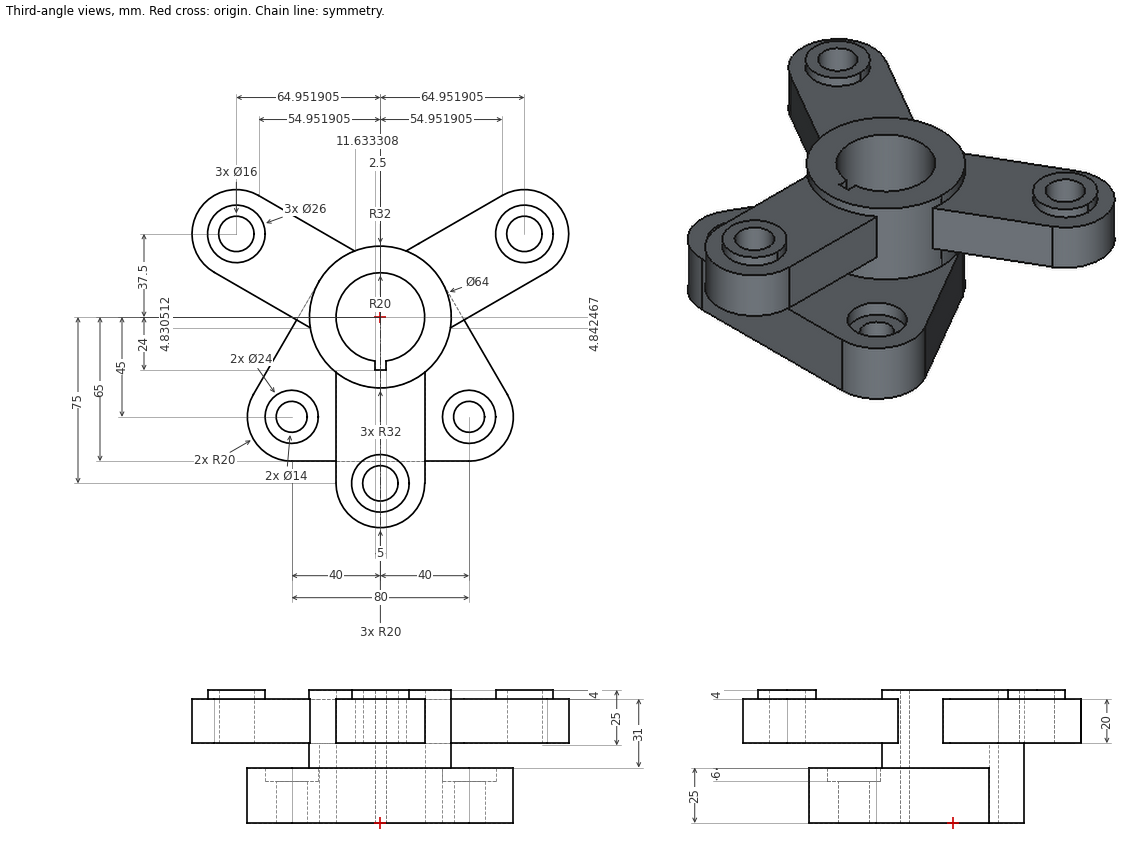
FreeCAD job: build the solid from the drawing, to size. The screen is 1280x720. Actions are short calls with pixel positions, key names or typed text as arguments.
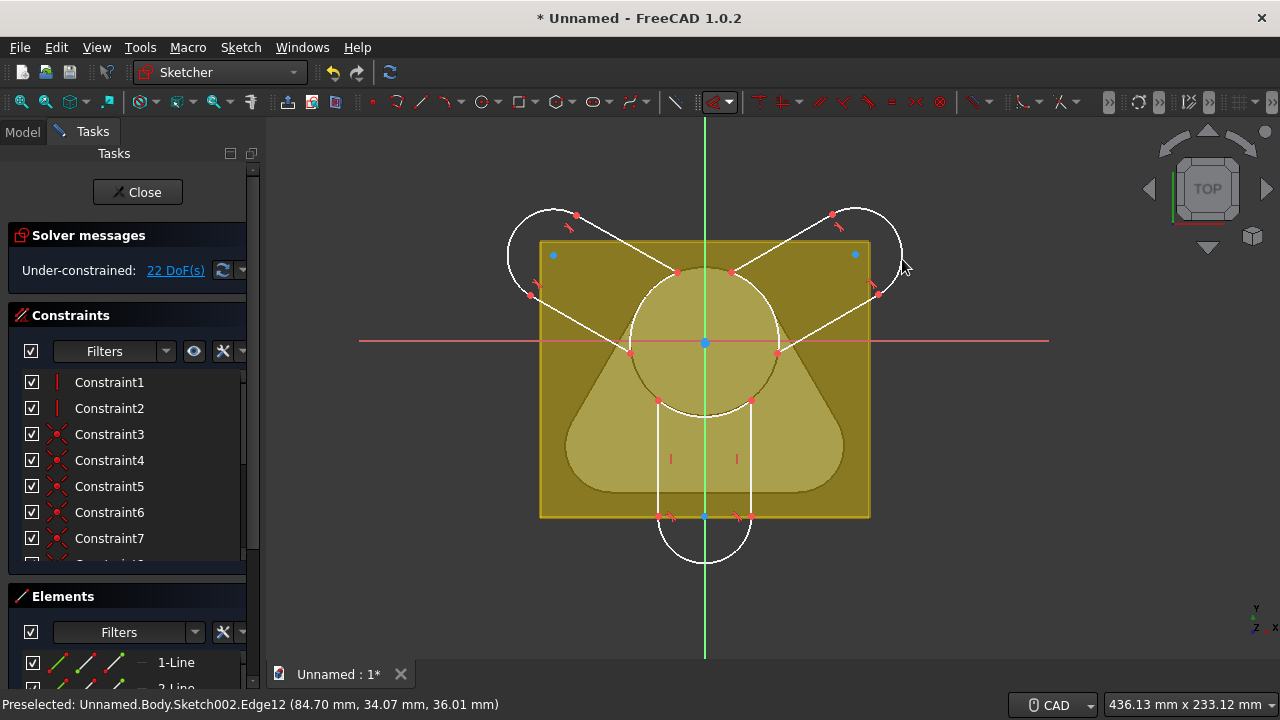
click(685, 414)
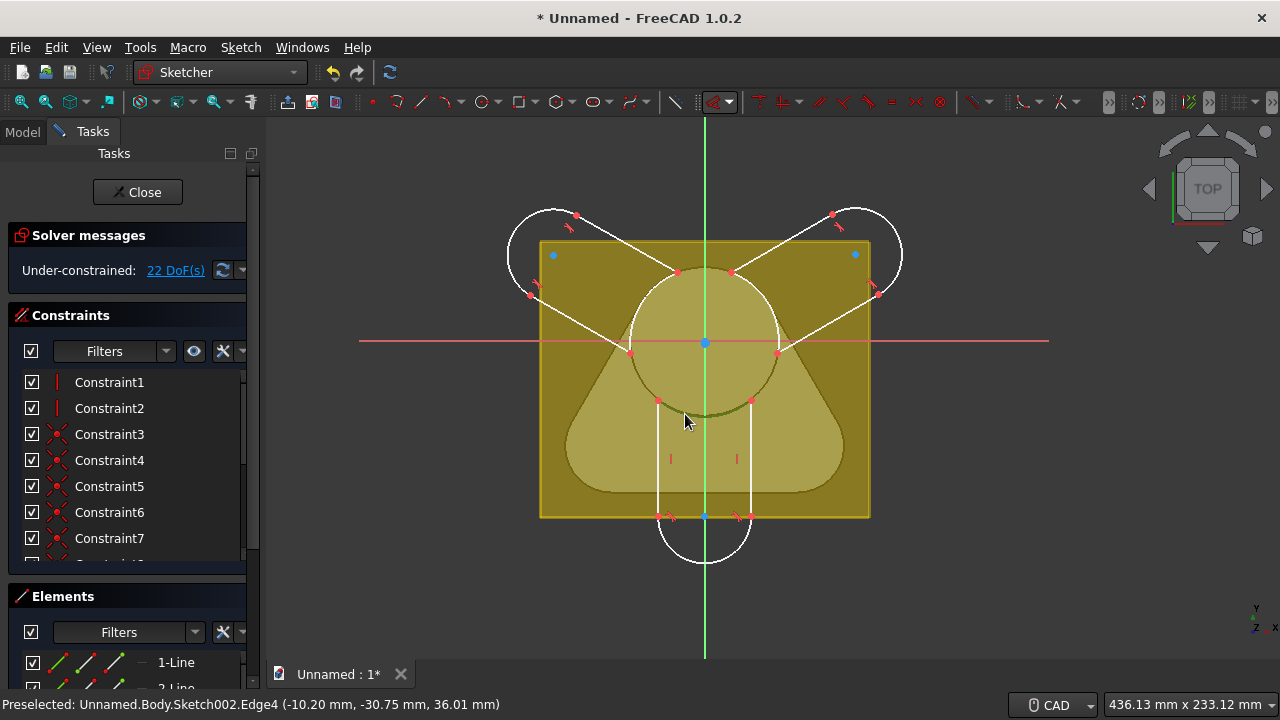
click(653, 289)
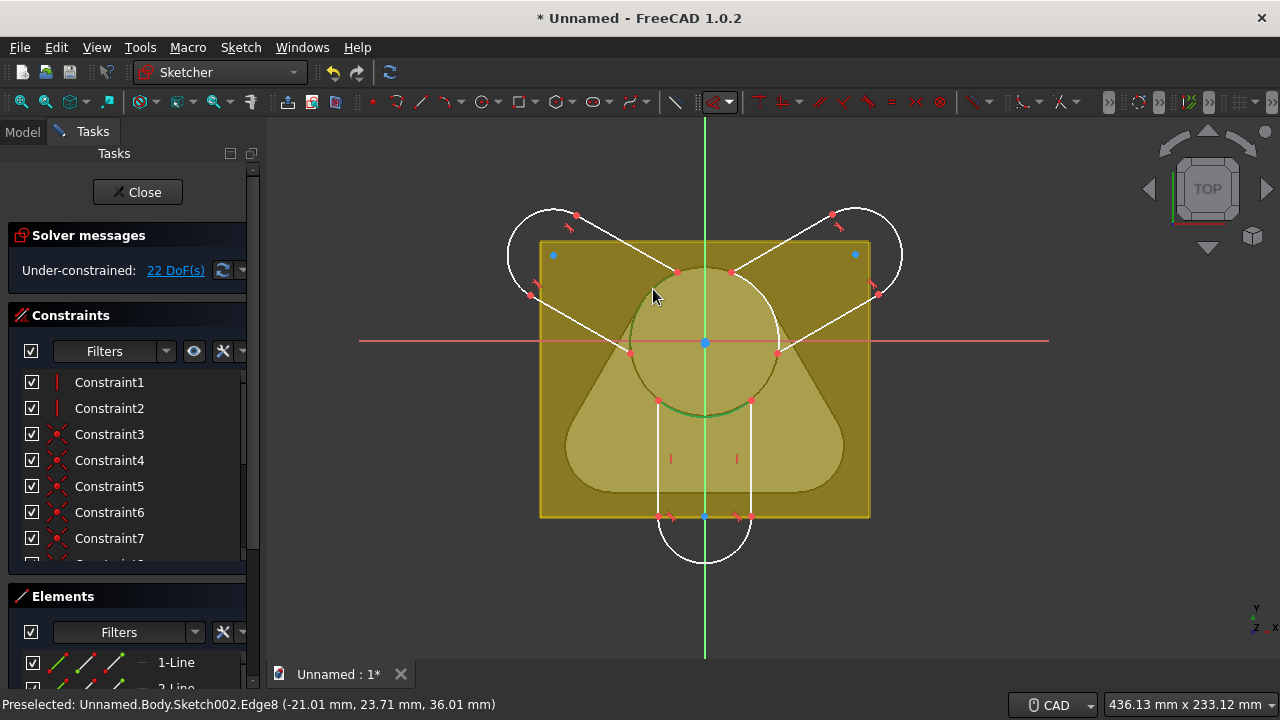
key(c)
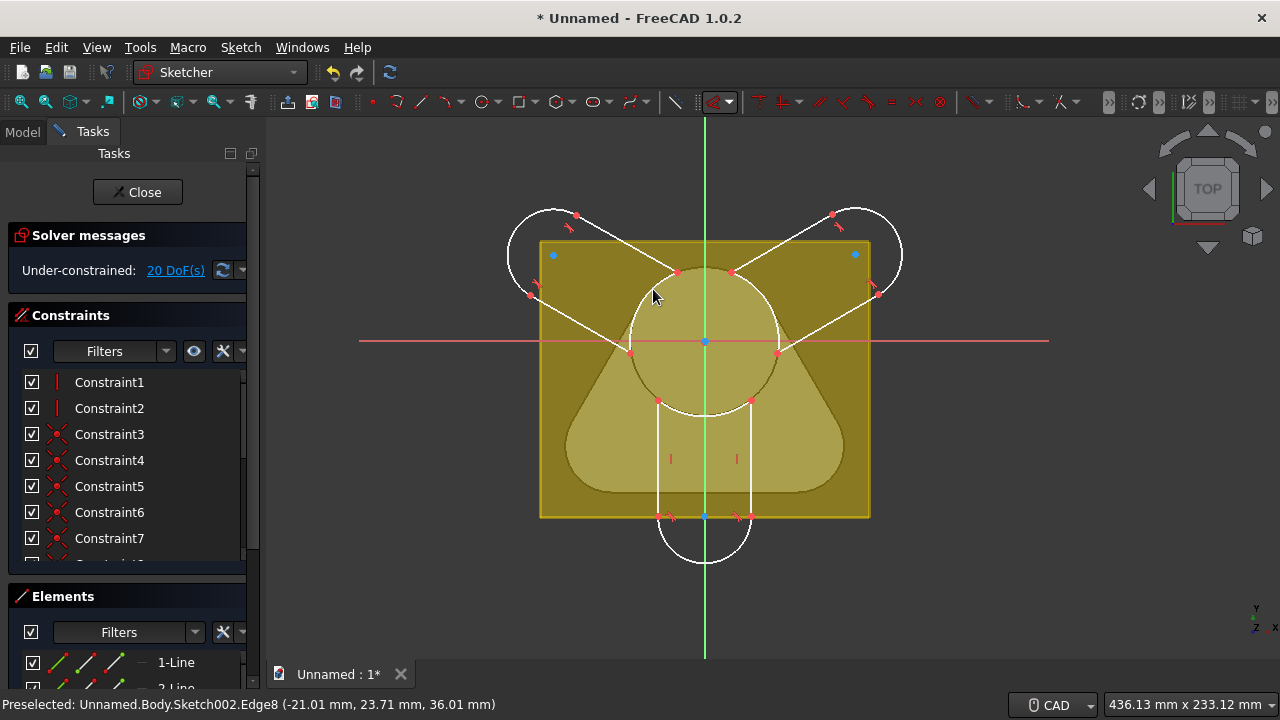
click(685, 414)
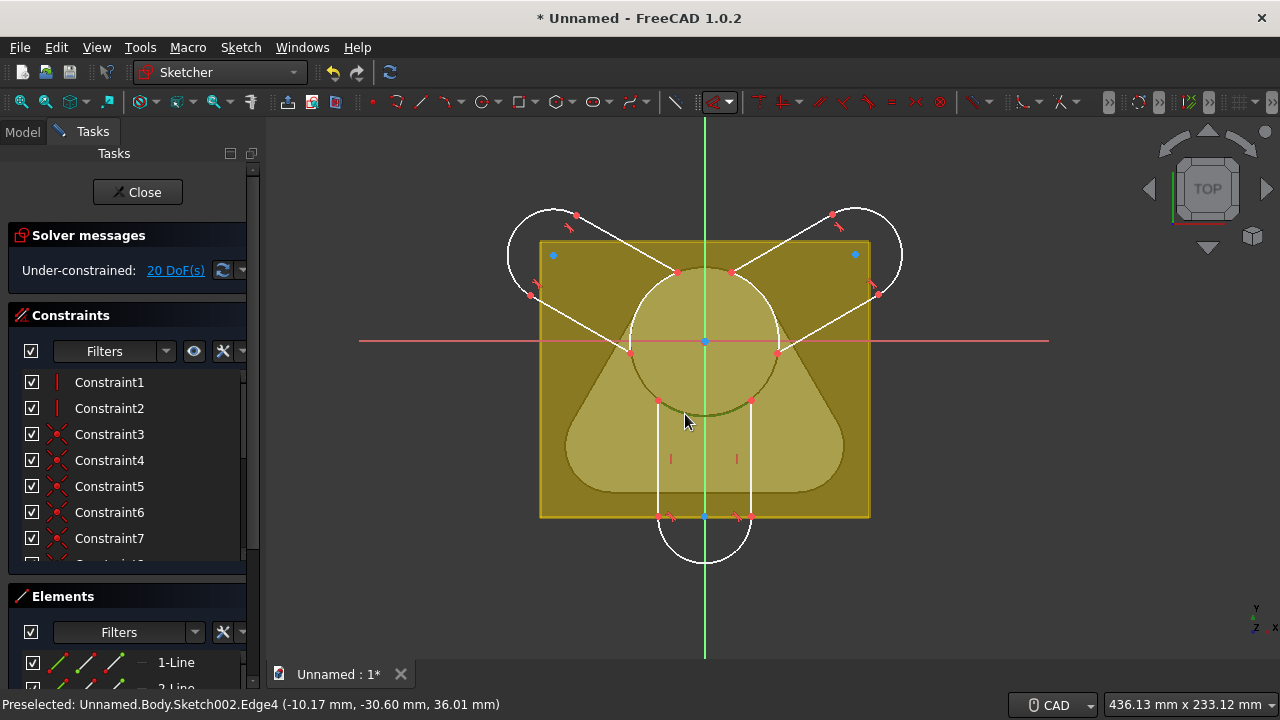
click(777, 323)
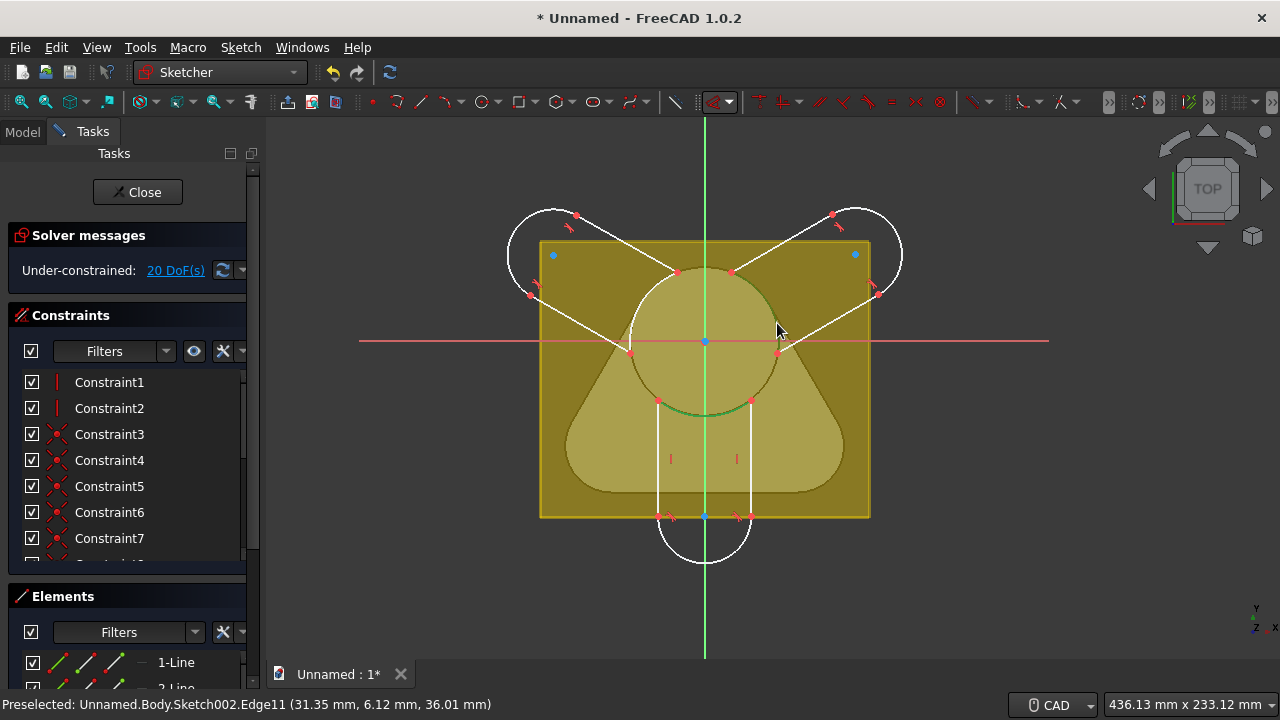
key(c)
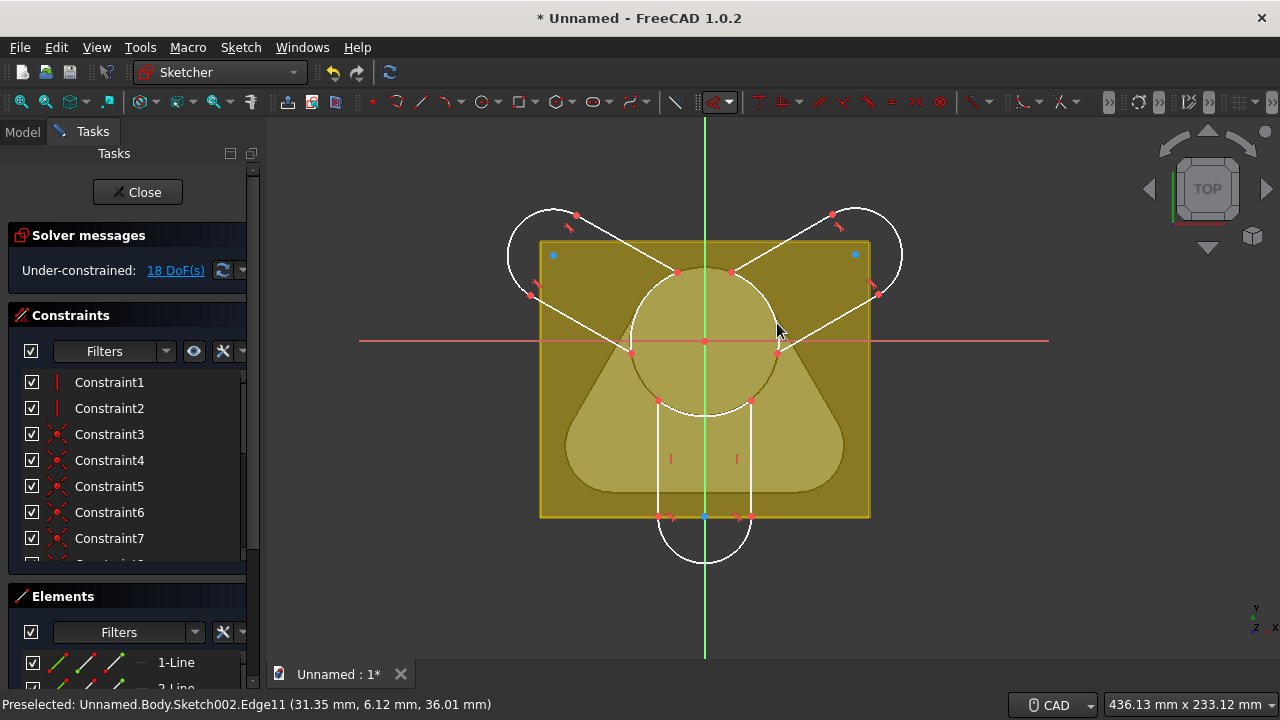
drag(695, 331, 715, 352)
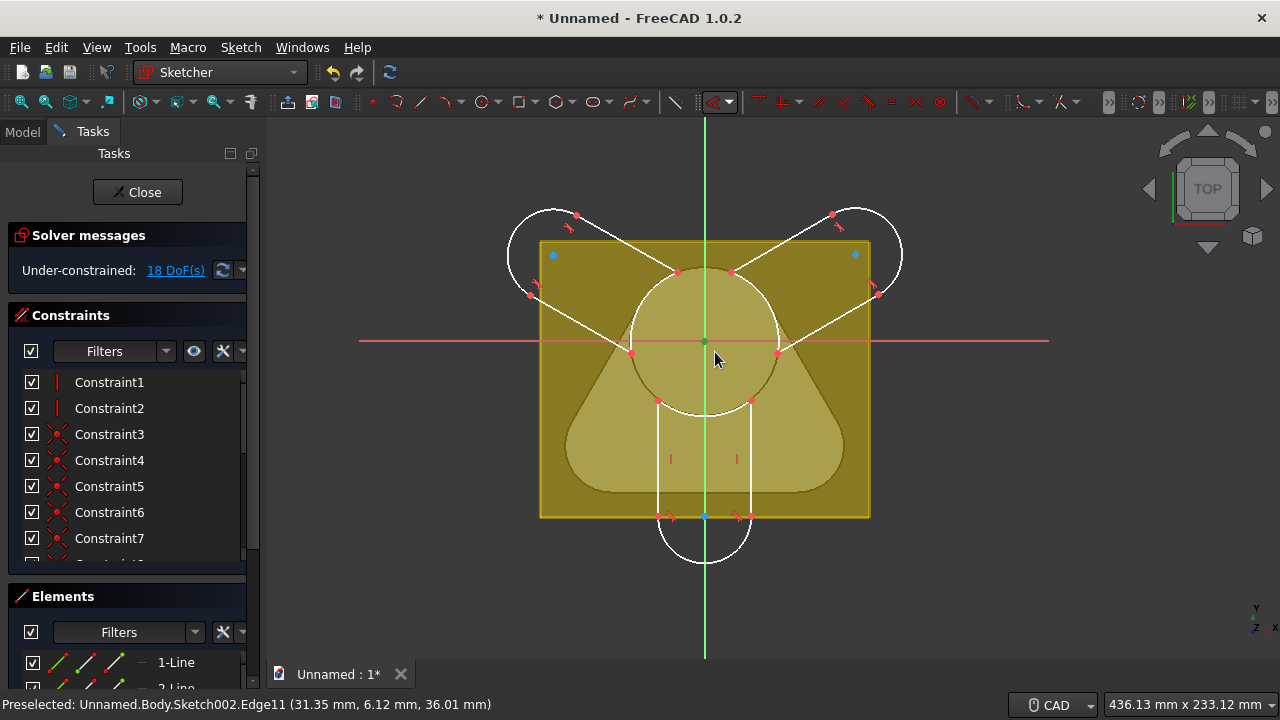
key(c)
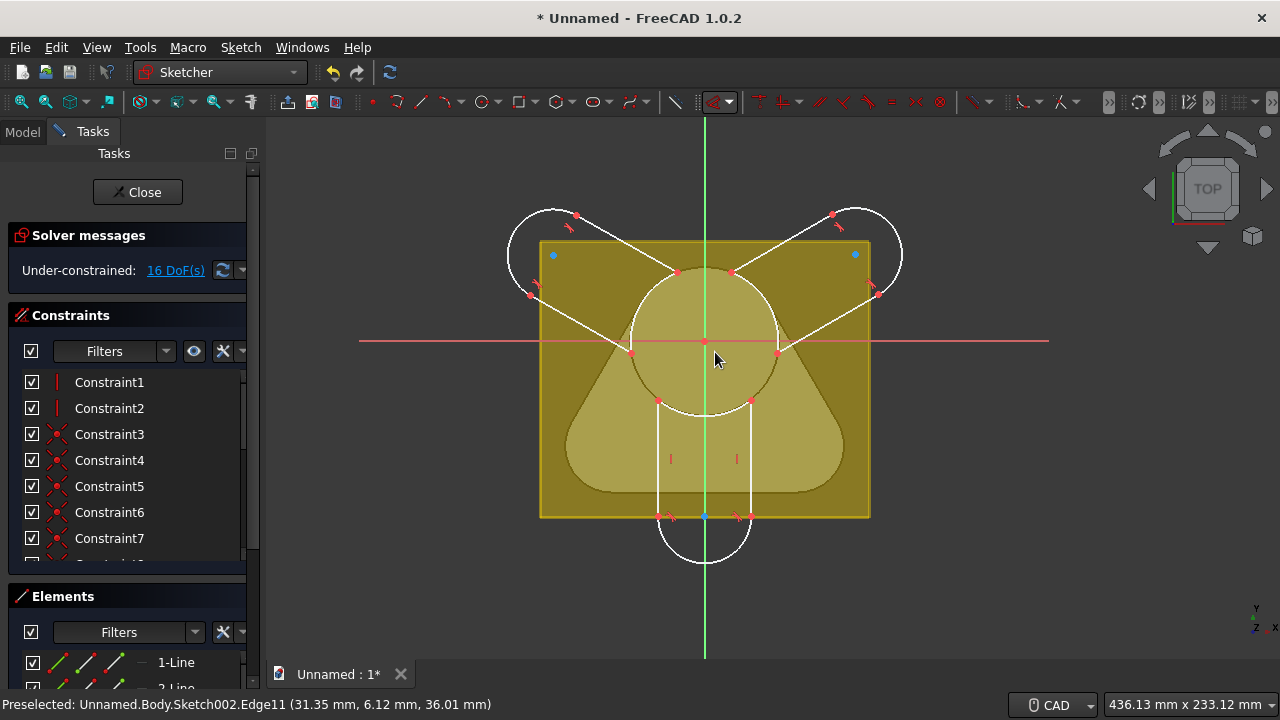
click(677, 554)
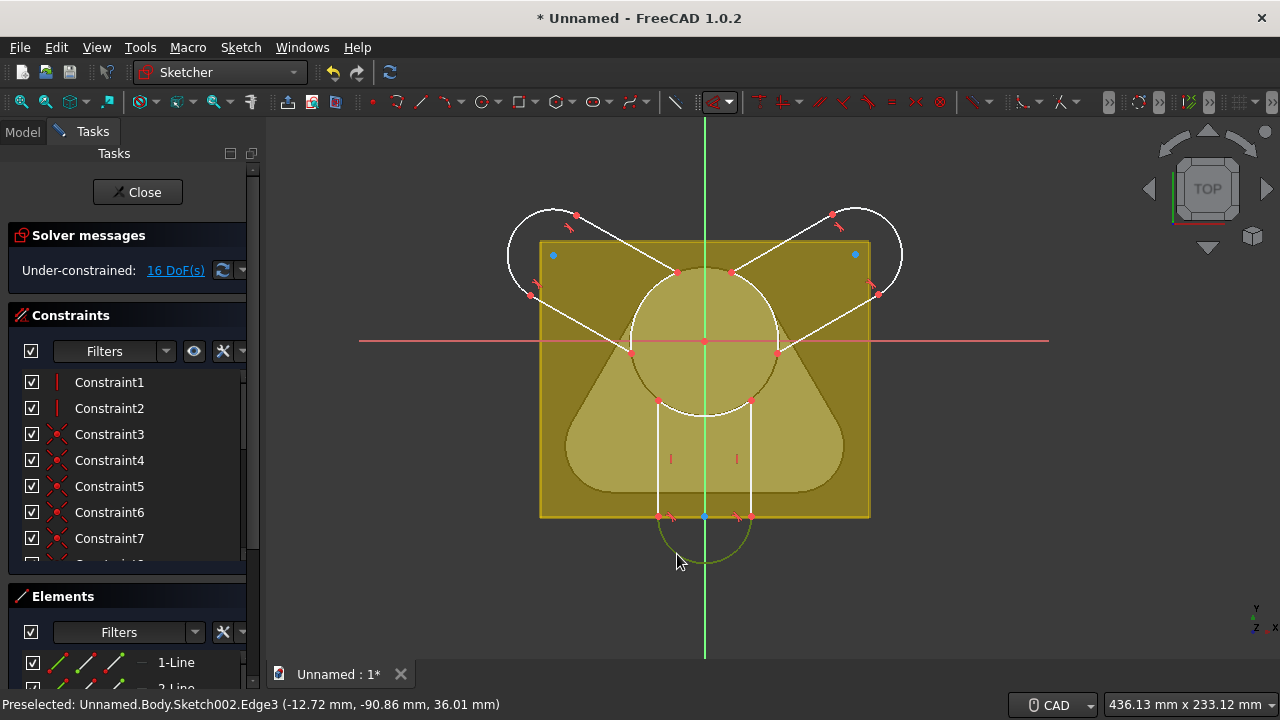
click(535, 214)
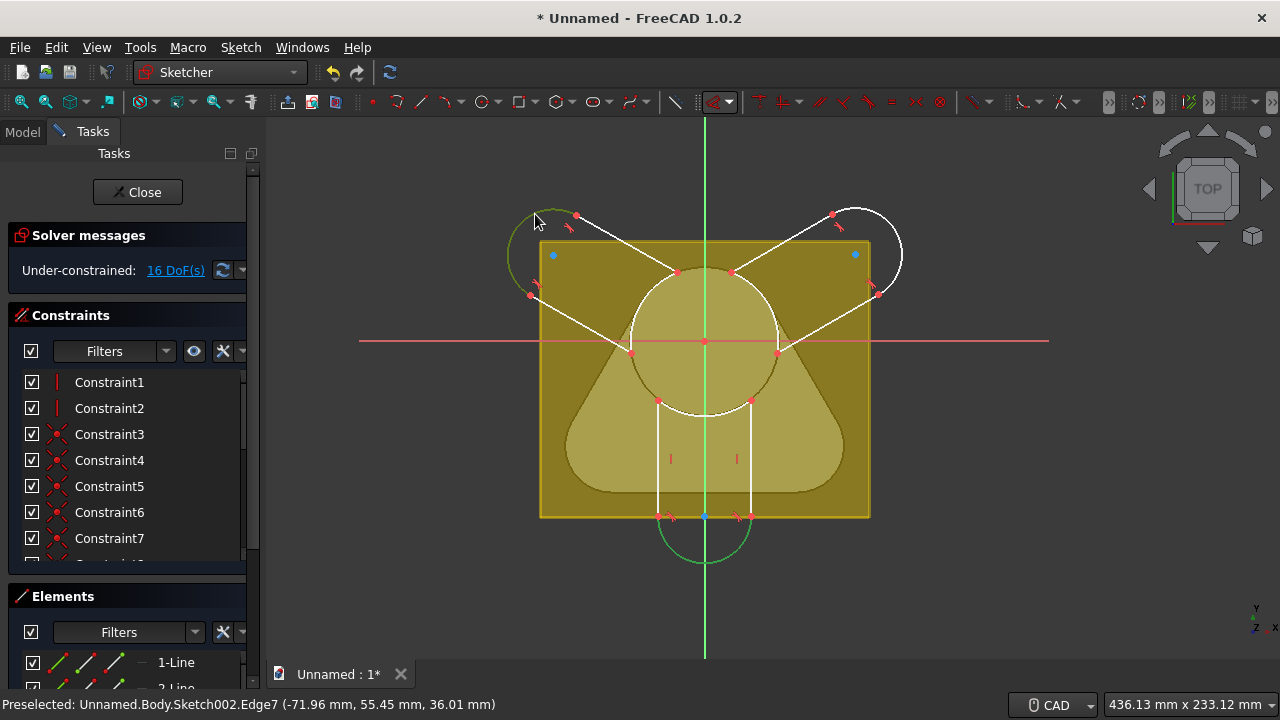
click(902, 259)